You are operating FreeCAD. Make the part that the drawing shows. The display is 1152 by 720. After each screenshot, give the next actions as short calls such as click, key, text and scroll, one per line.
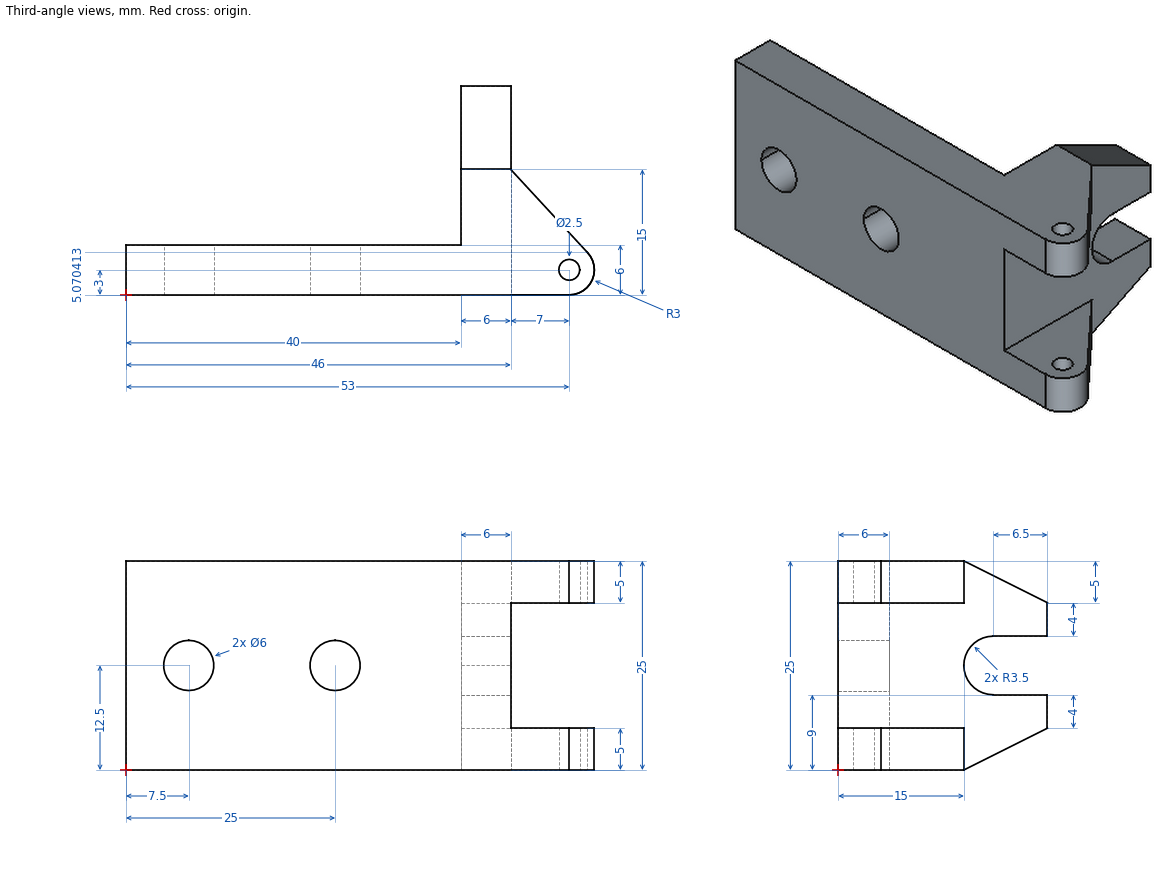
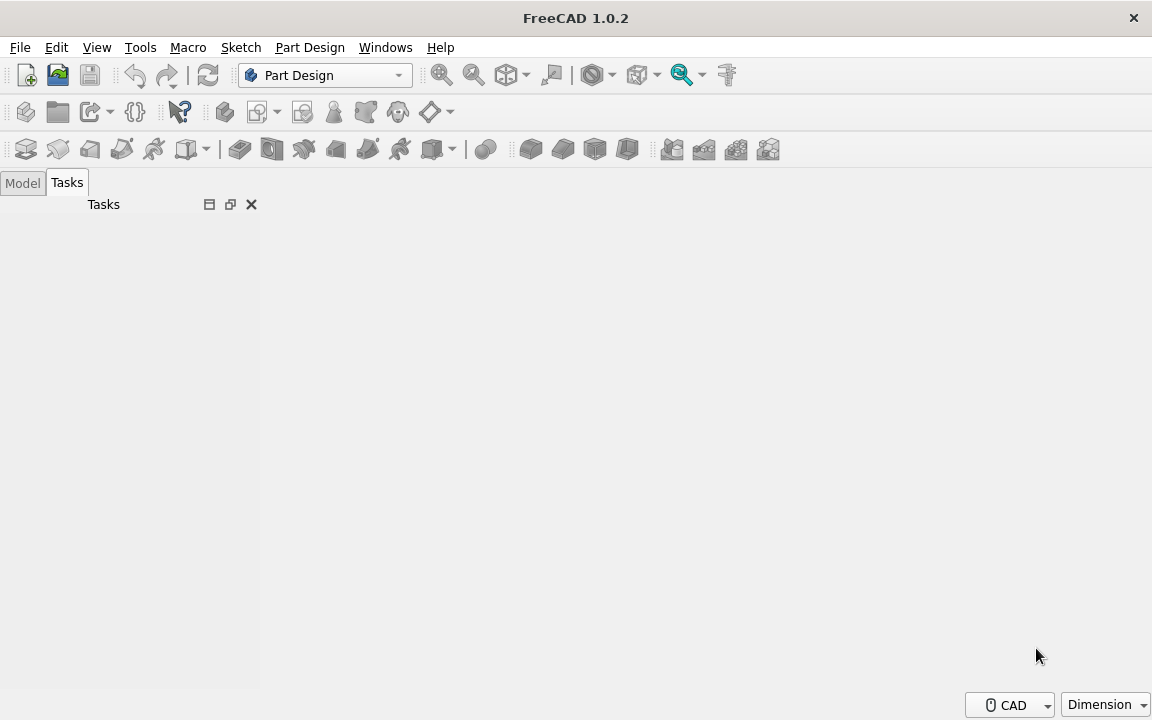
key(ctrl+n)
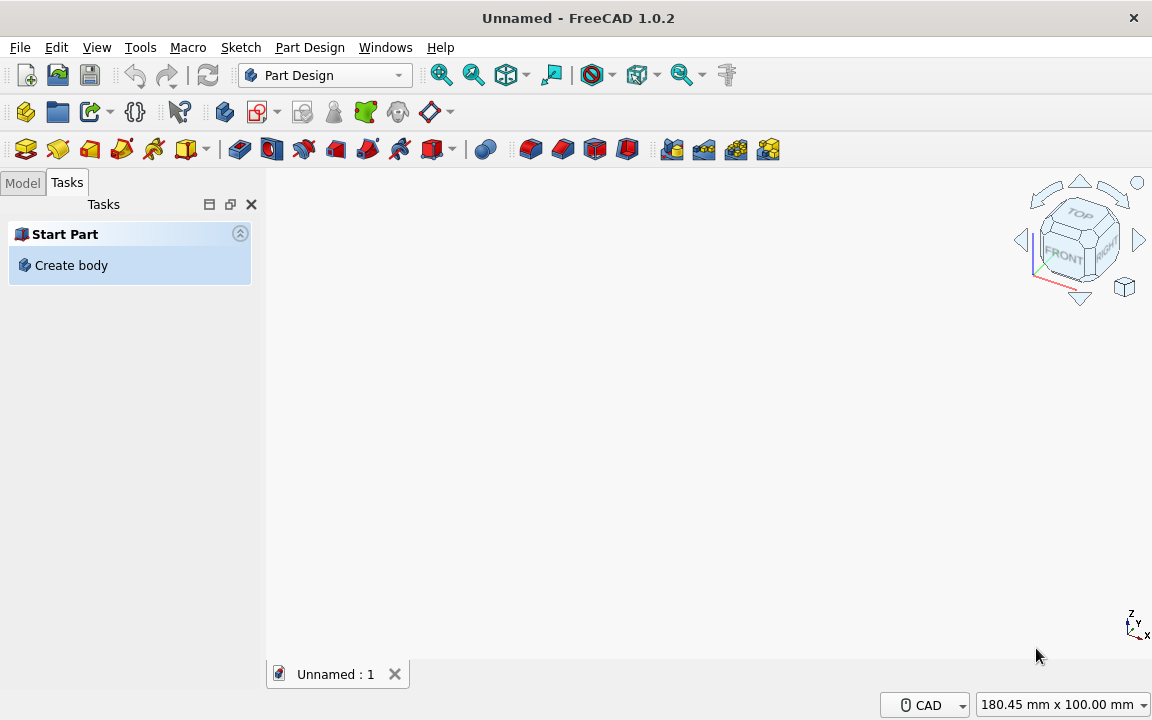
click(258, 112)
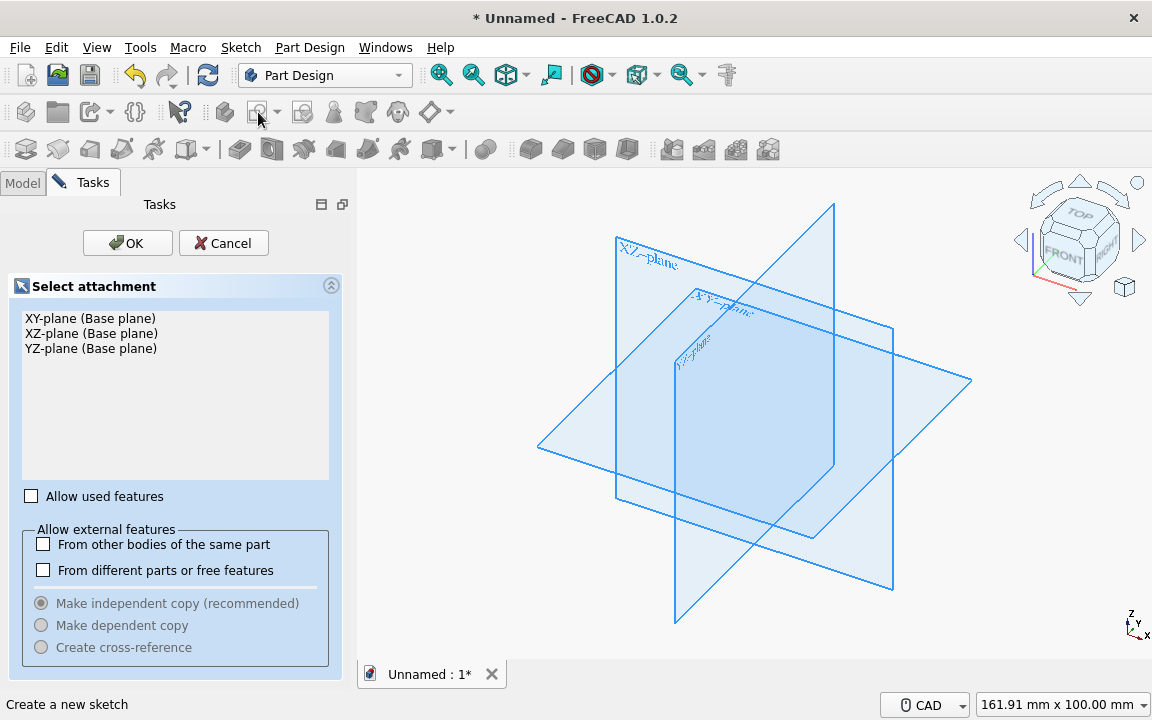
click(82, 318)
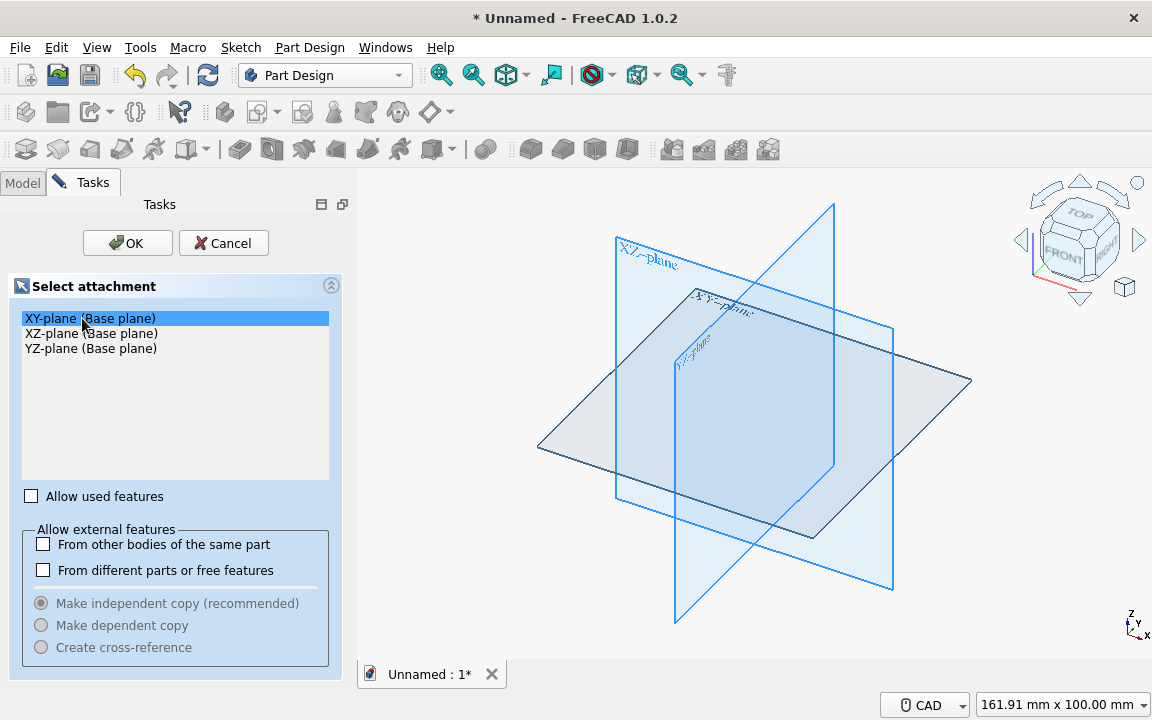
click(128, 243)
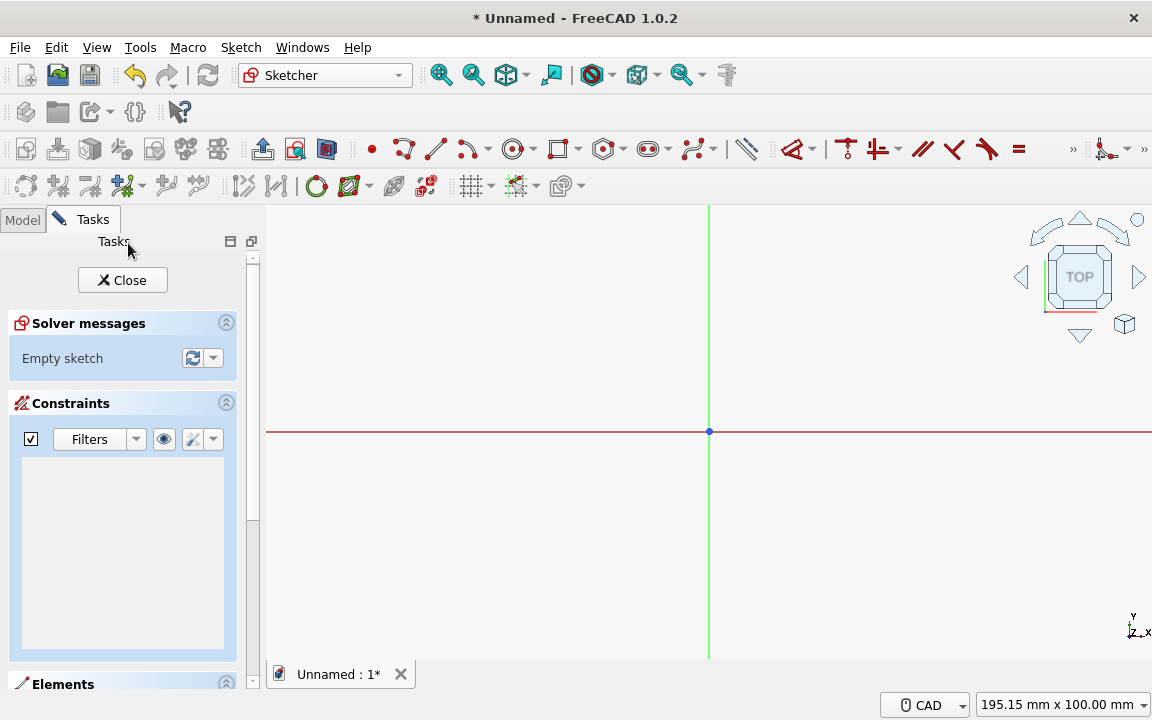
scroll(893, 410, up, 5)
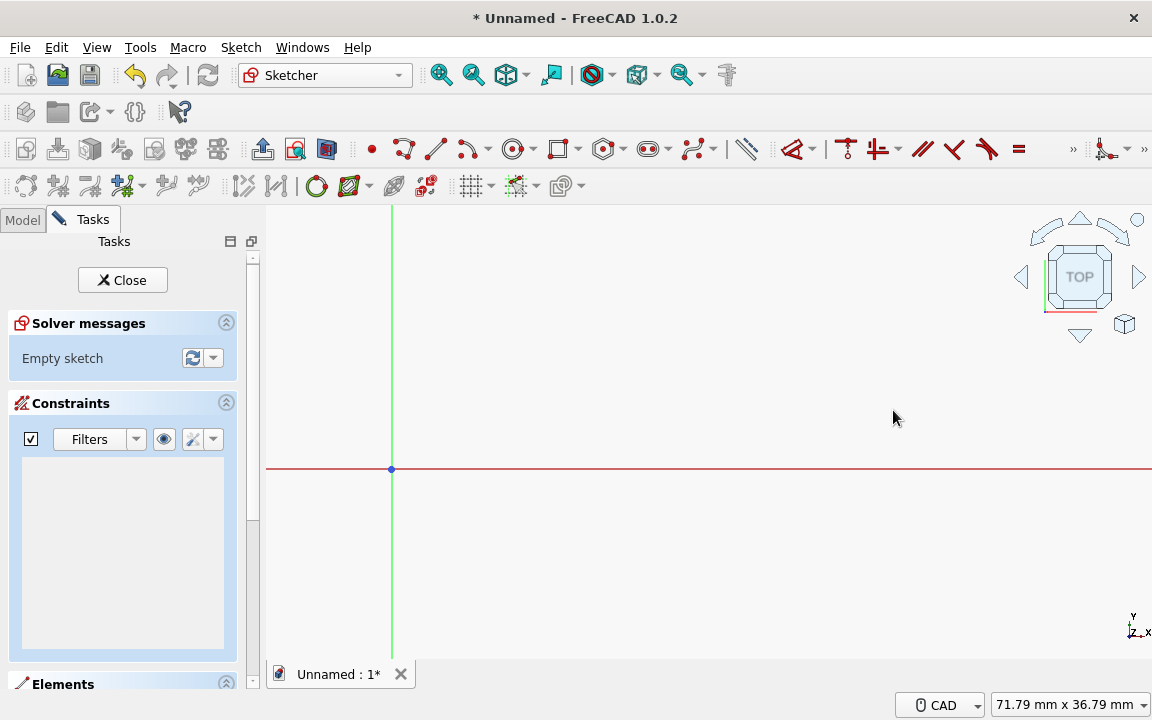
key(g)
key(r)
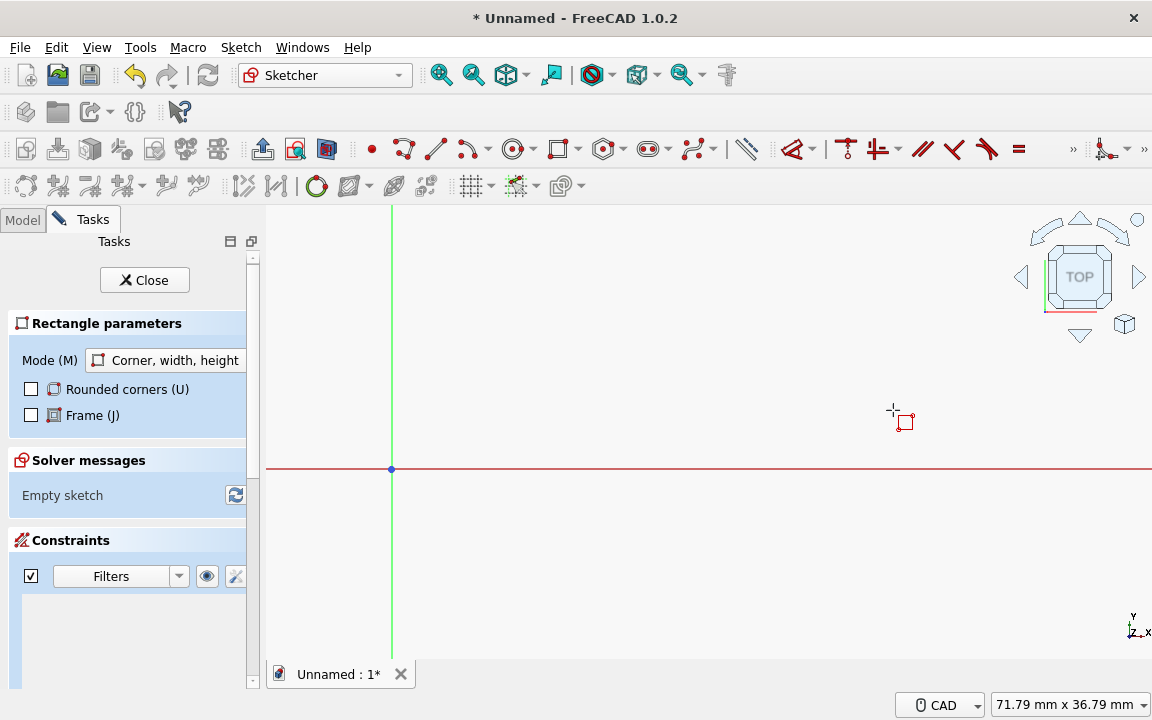
click(392, 469)
click(885, 395)
key(Escape)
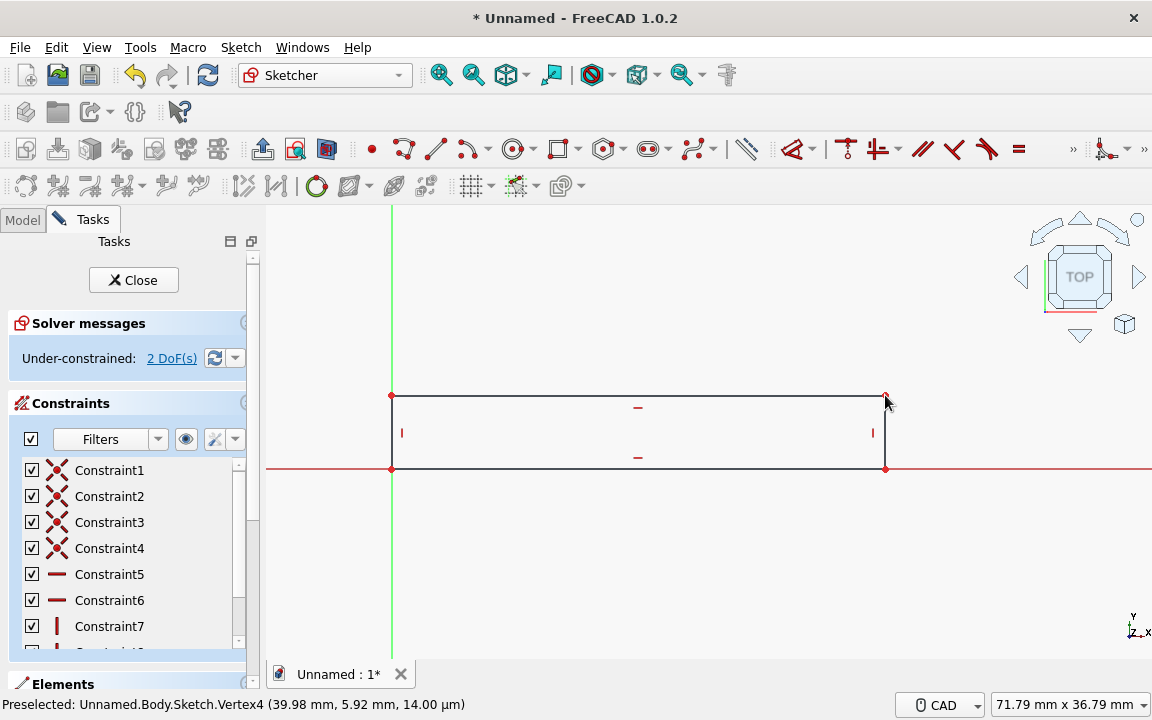
key(d)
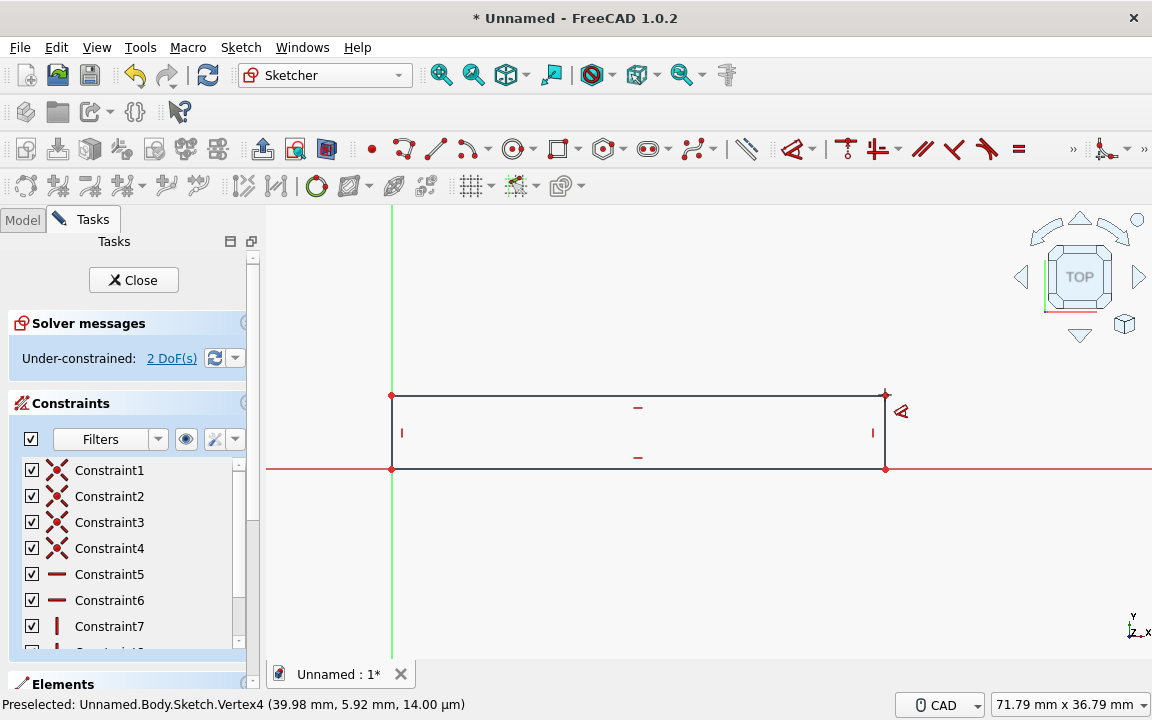
click(885, 447)
click(919, 433)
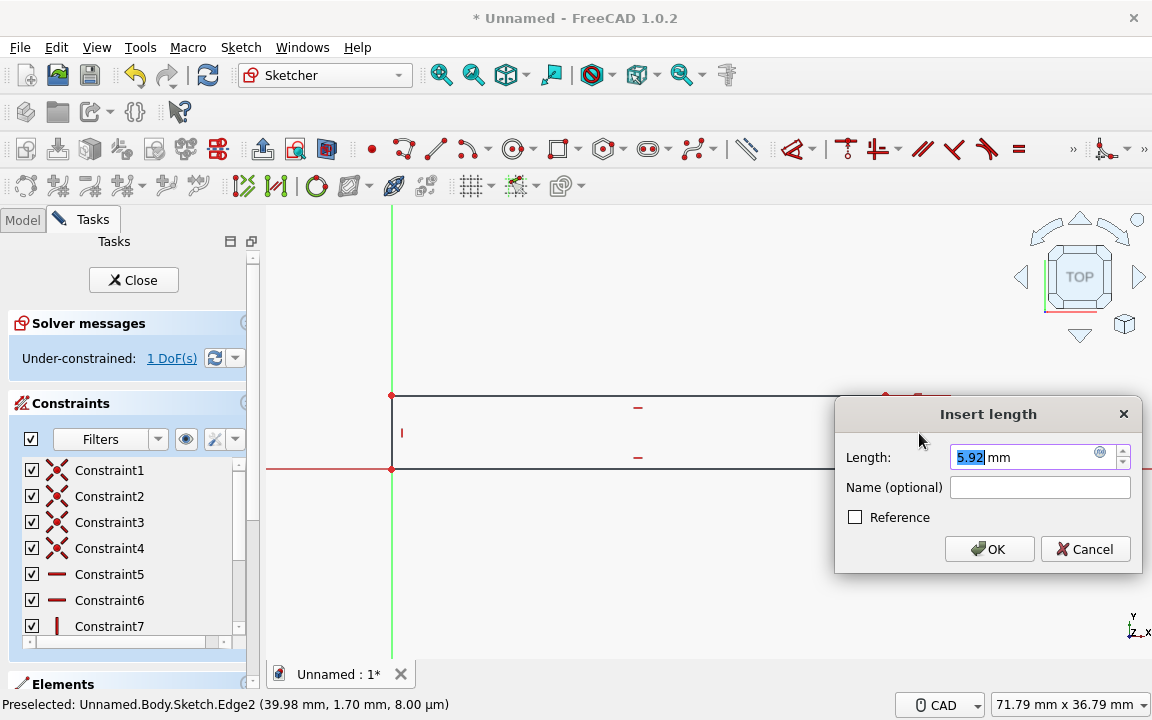
text(6)
key(Return)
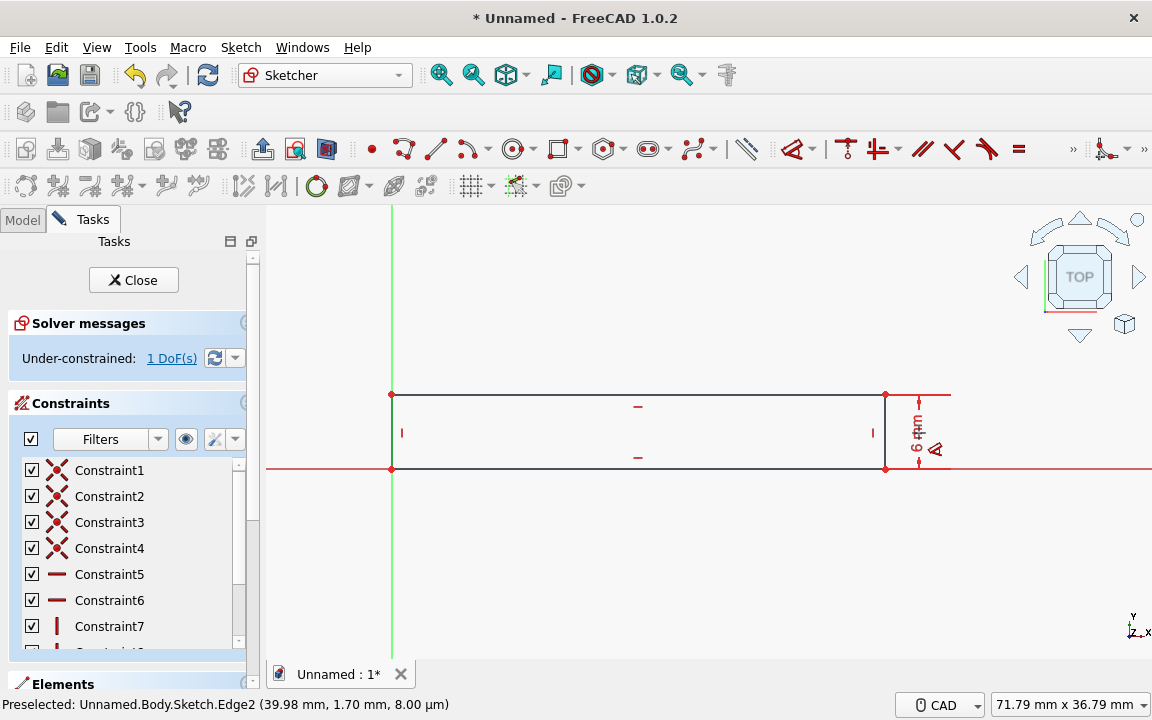
click(540, 469)
click(638, 503)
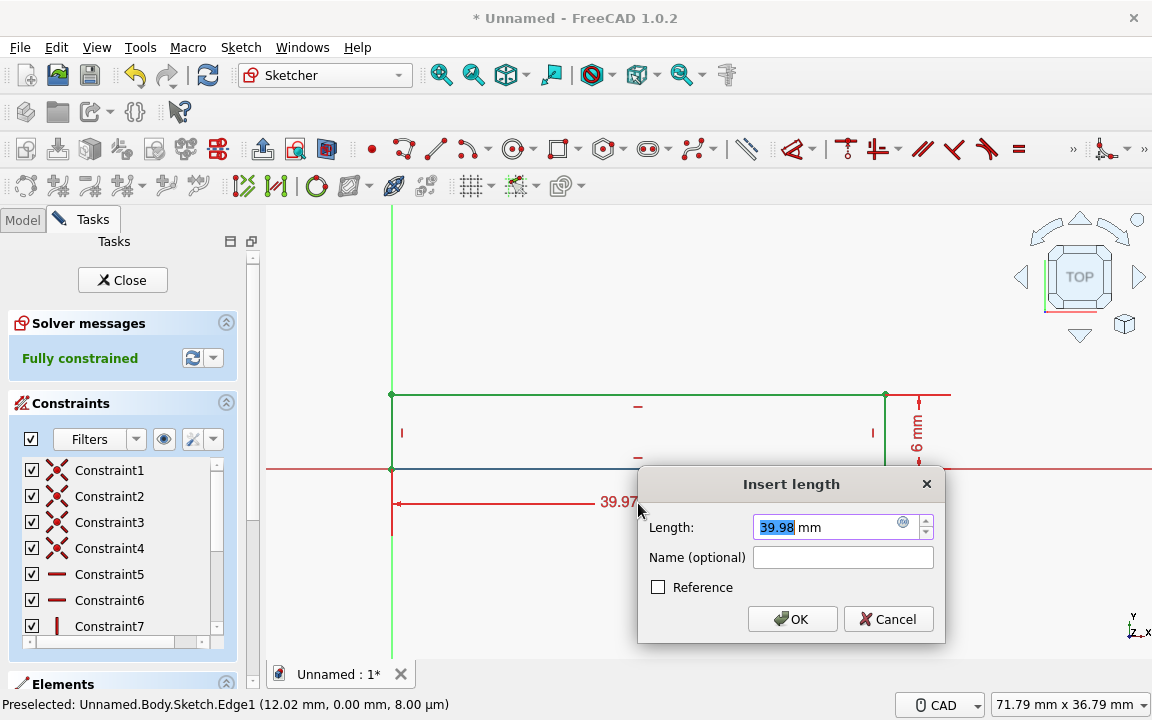
text(40)
key(Return)
key(Escape)